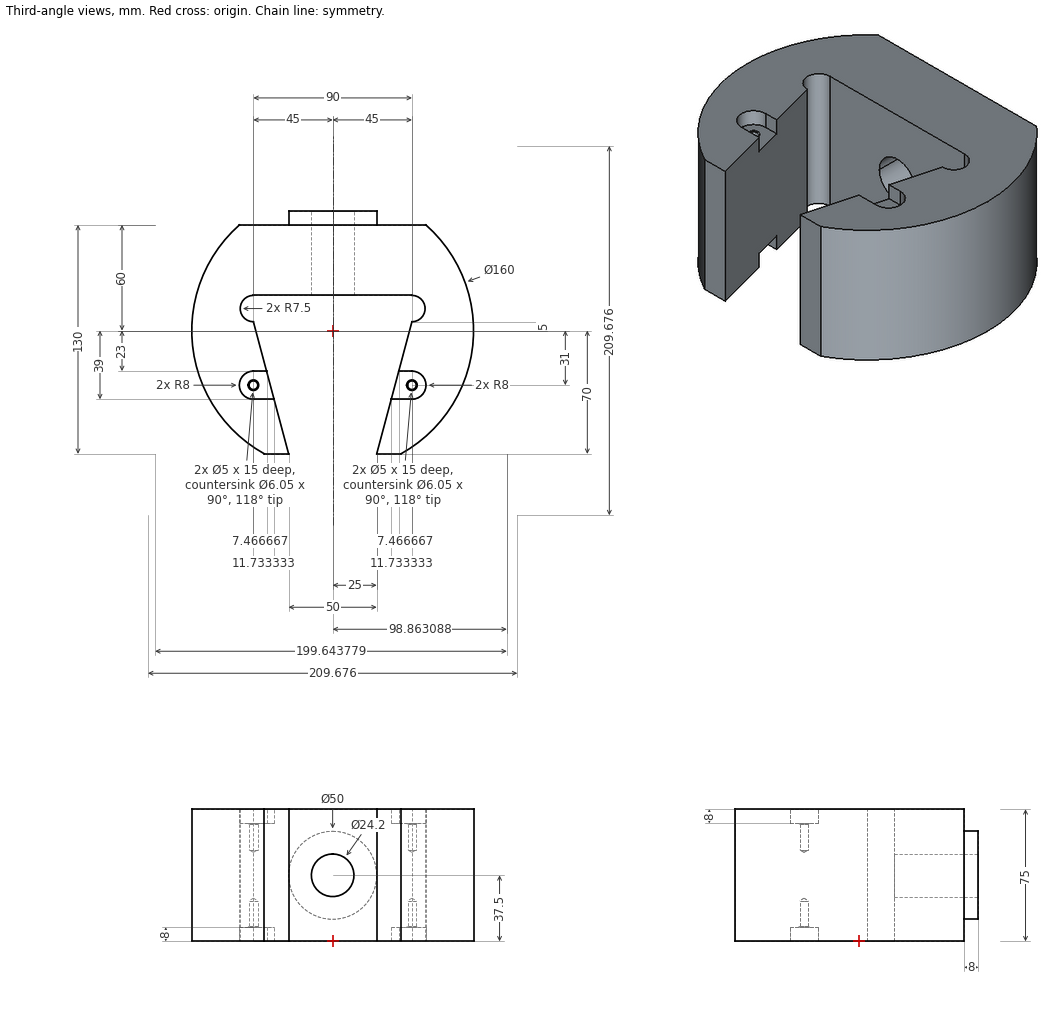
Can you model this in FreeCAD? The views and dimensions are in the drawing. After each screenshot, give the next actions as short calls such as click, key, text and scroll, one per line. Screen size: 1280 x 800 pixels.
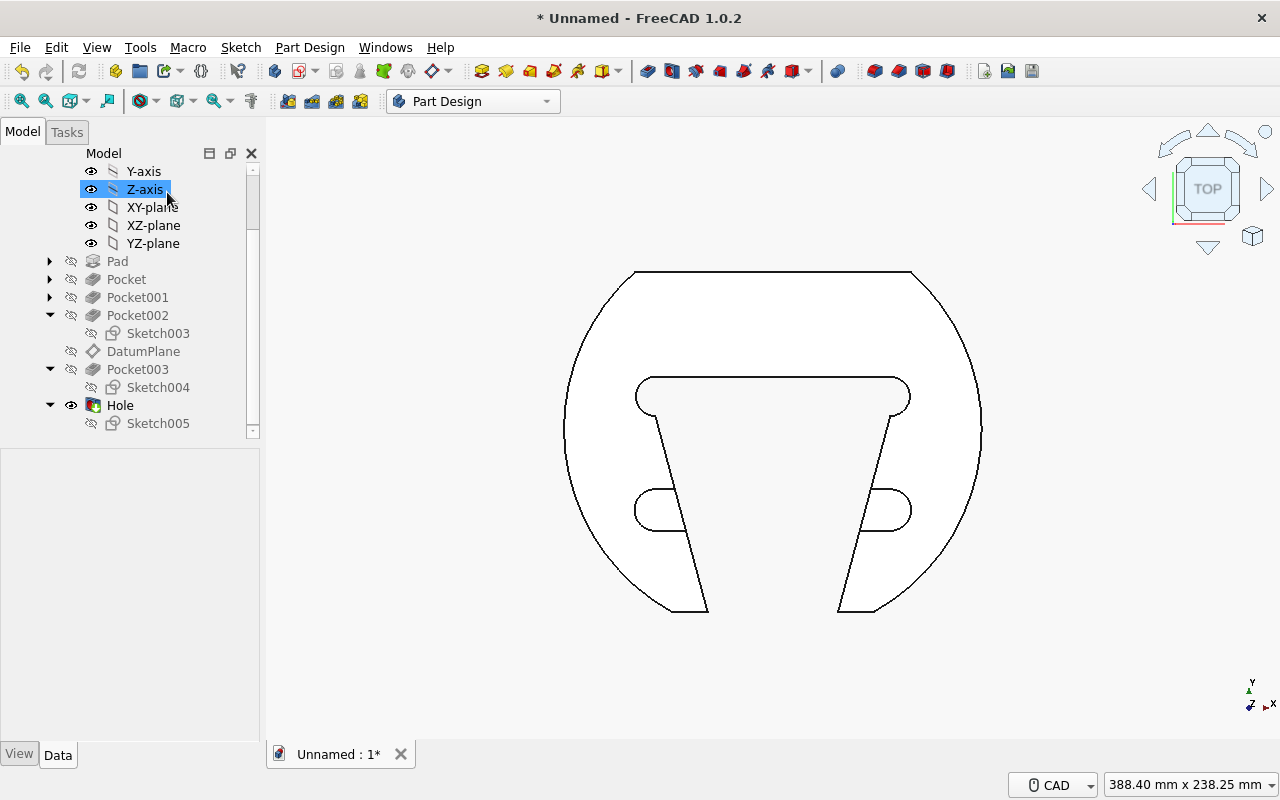
click(660, 509)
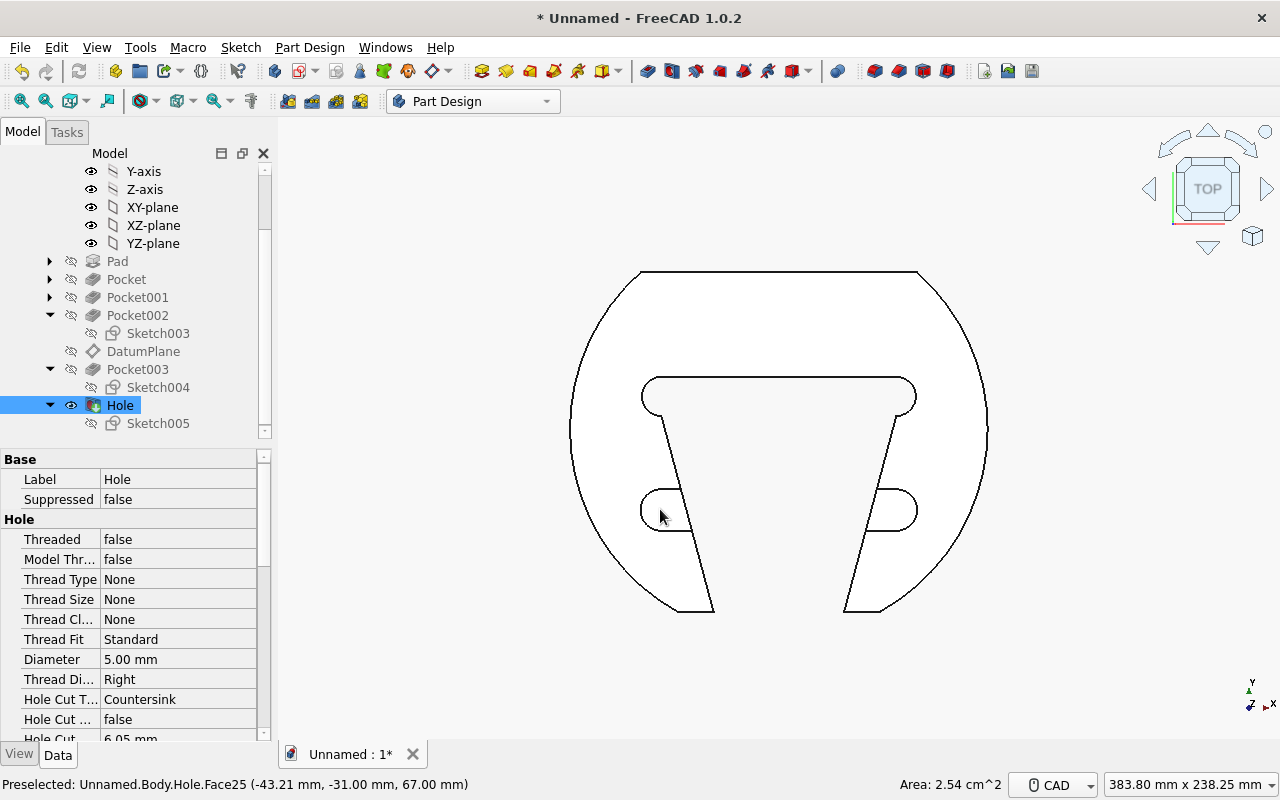
click(300, 72)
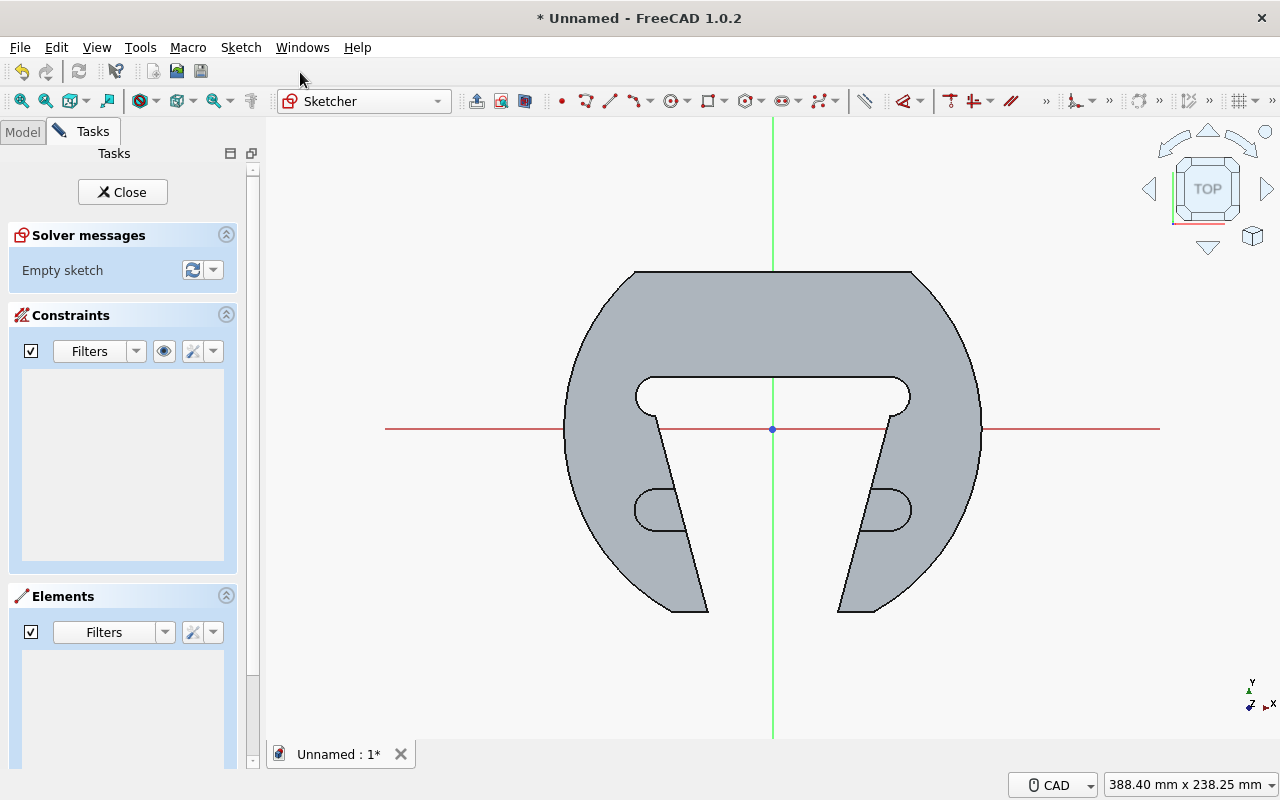
key(q)
key(s)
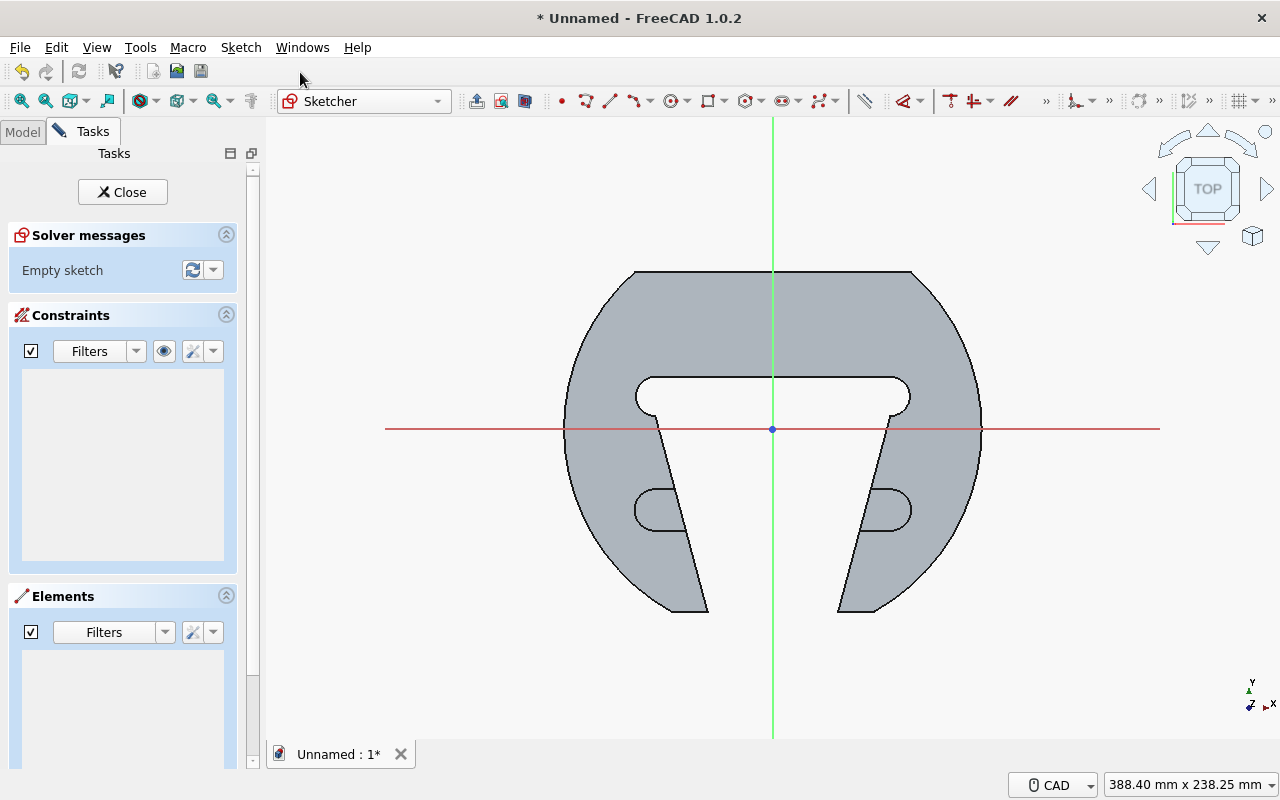
scroll(829, 509, up, 4)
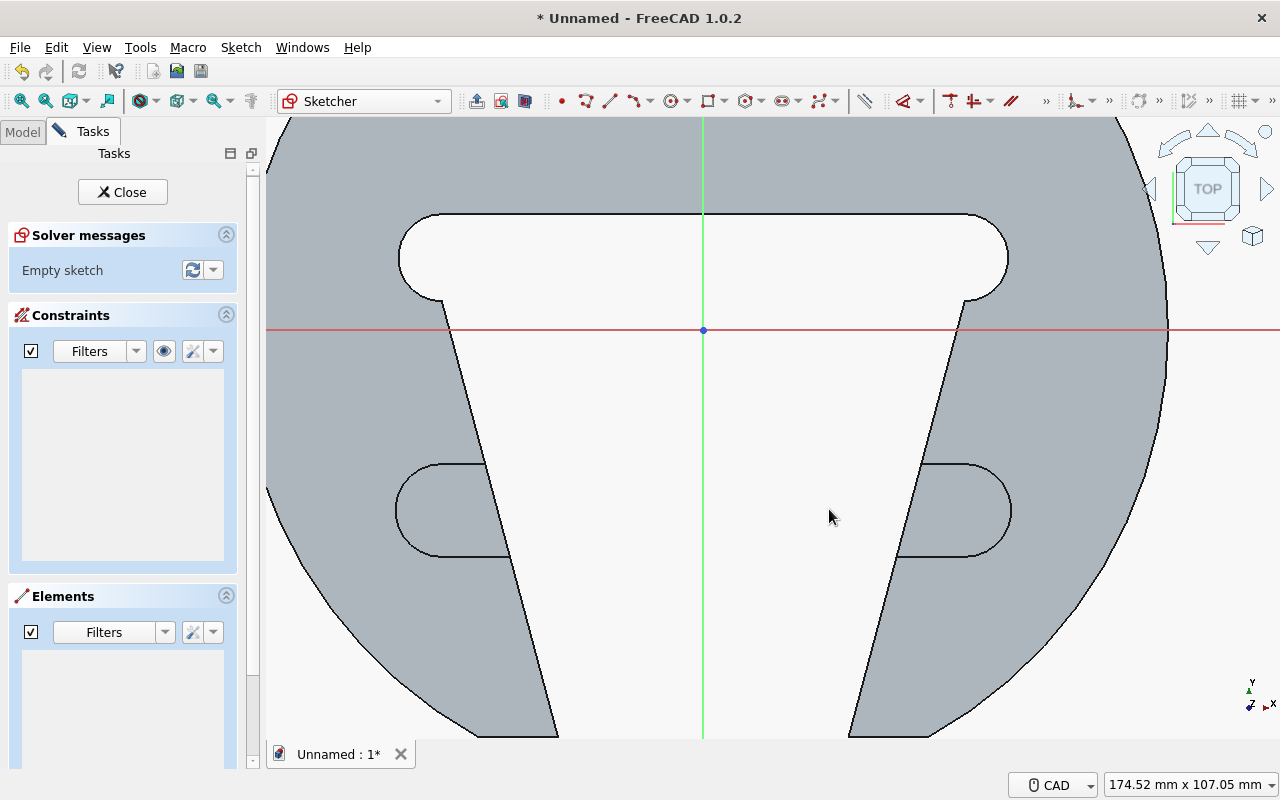
click(672, 102)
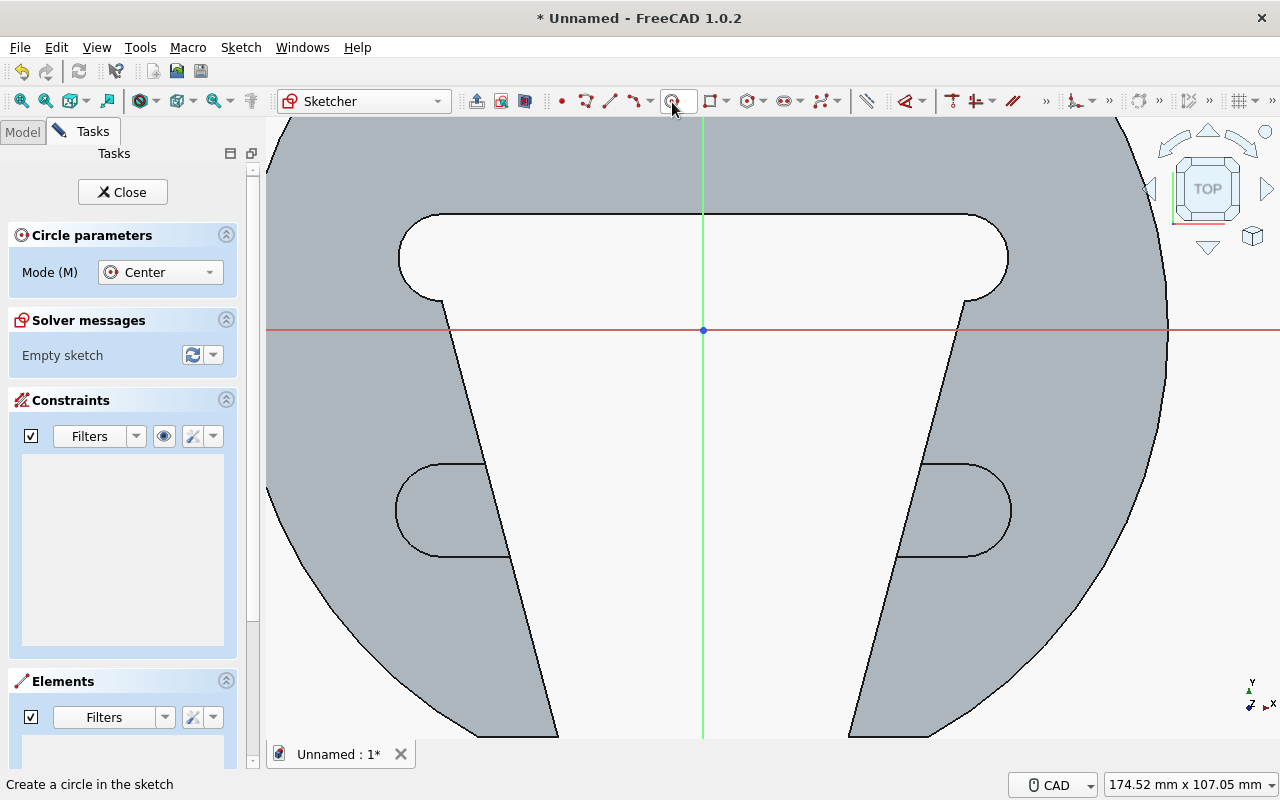
scroll(442, 510, up, 3)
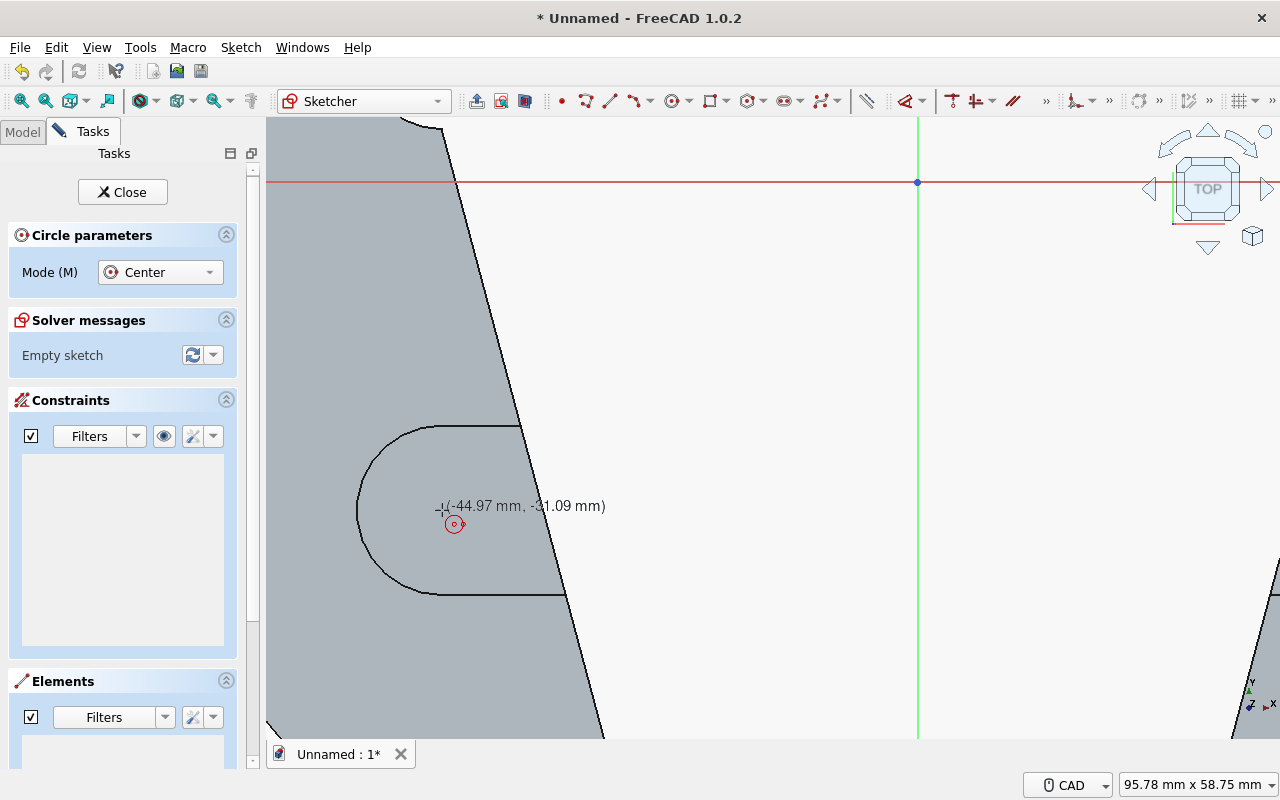
click(442, 510)
move(460, 492)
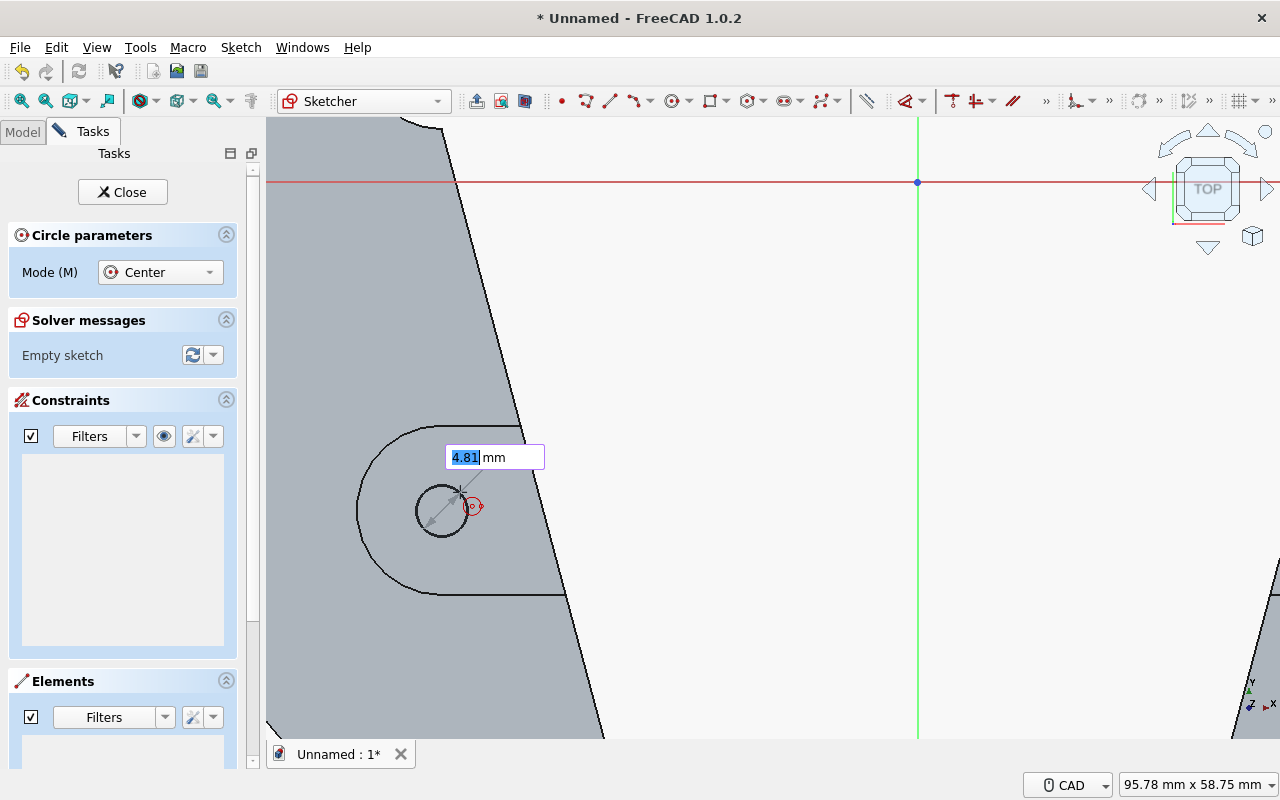
text(5)
key(Return)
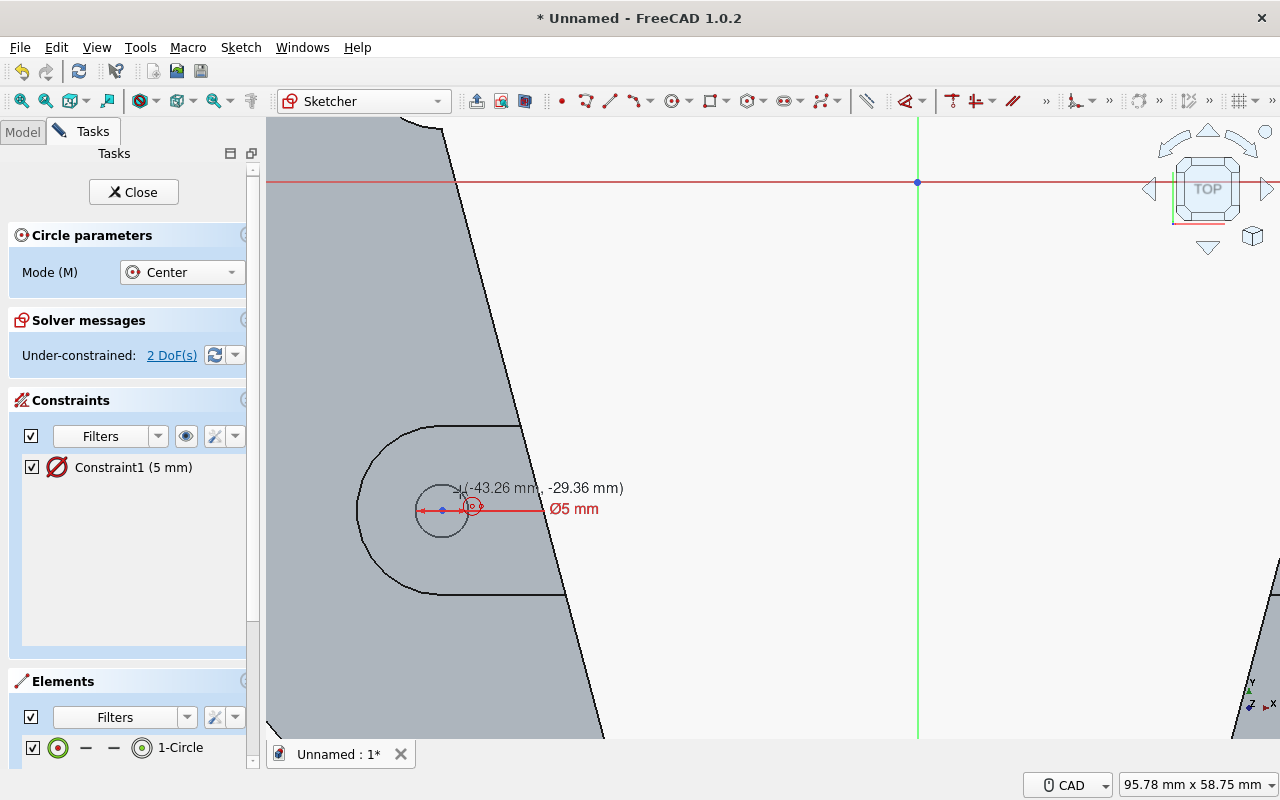
scroll(445, 511, down, 3)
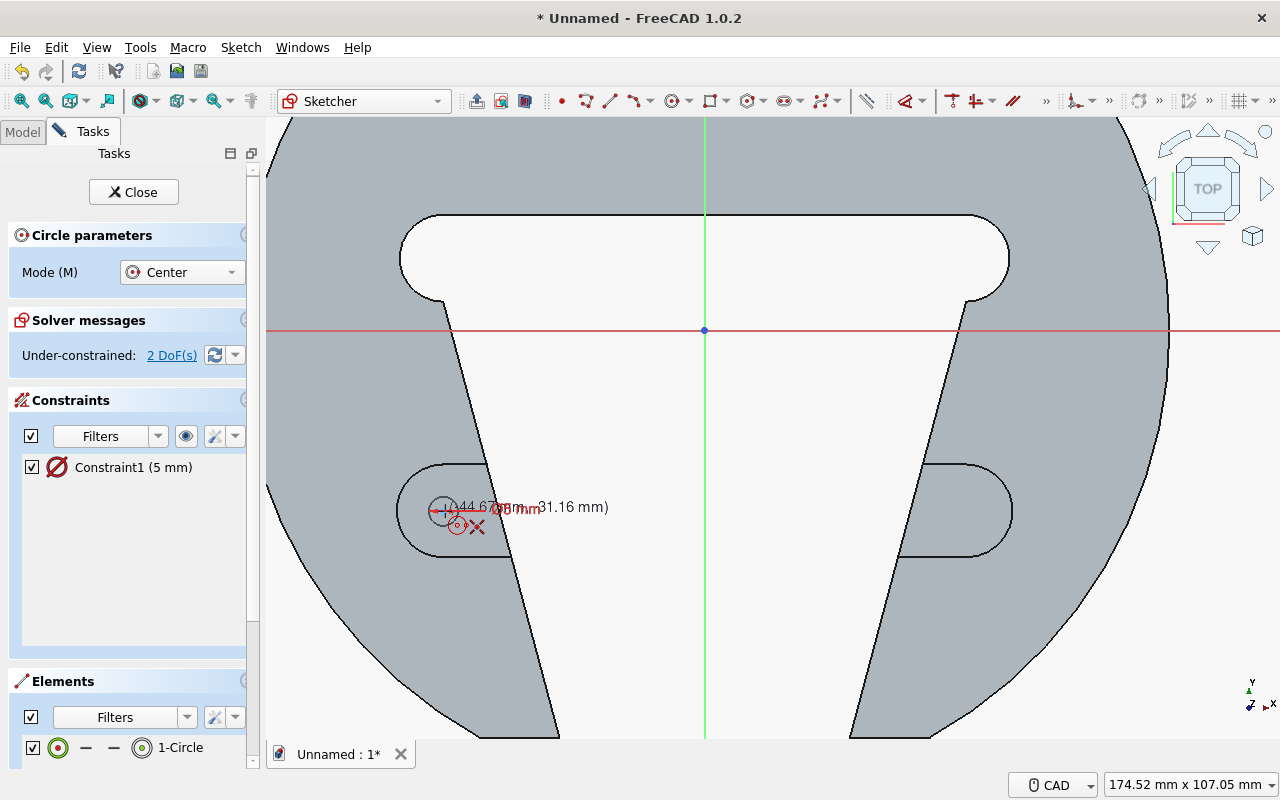
scroll(966, 511, up, 3)